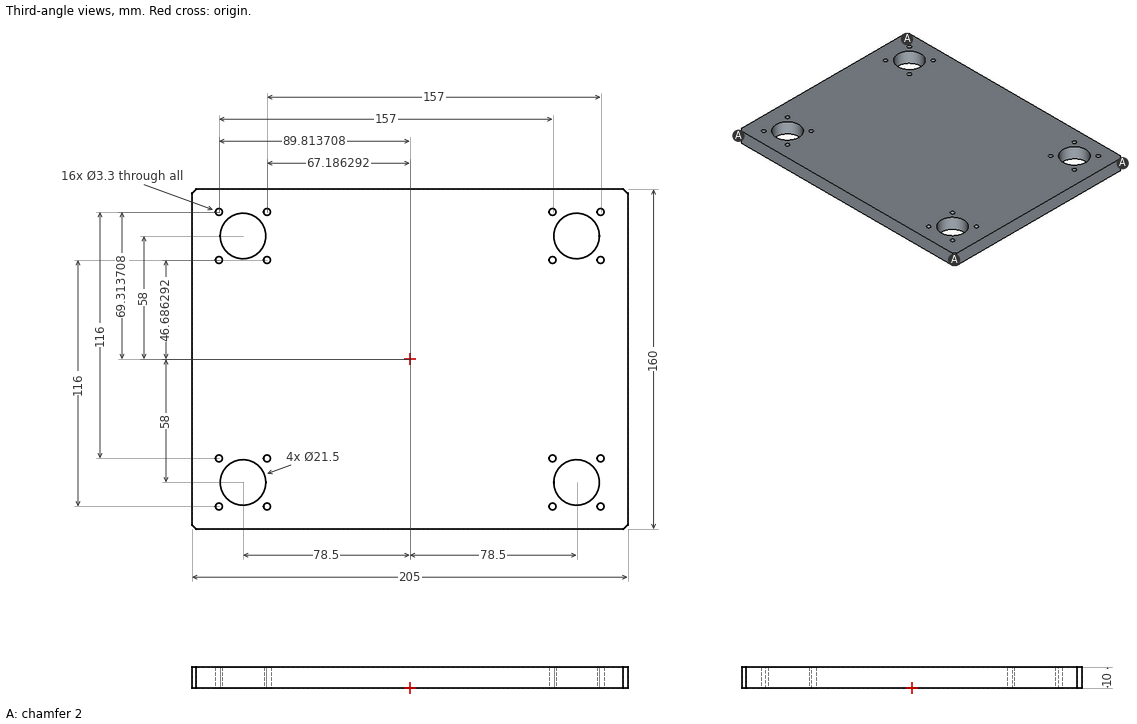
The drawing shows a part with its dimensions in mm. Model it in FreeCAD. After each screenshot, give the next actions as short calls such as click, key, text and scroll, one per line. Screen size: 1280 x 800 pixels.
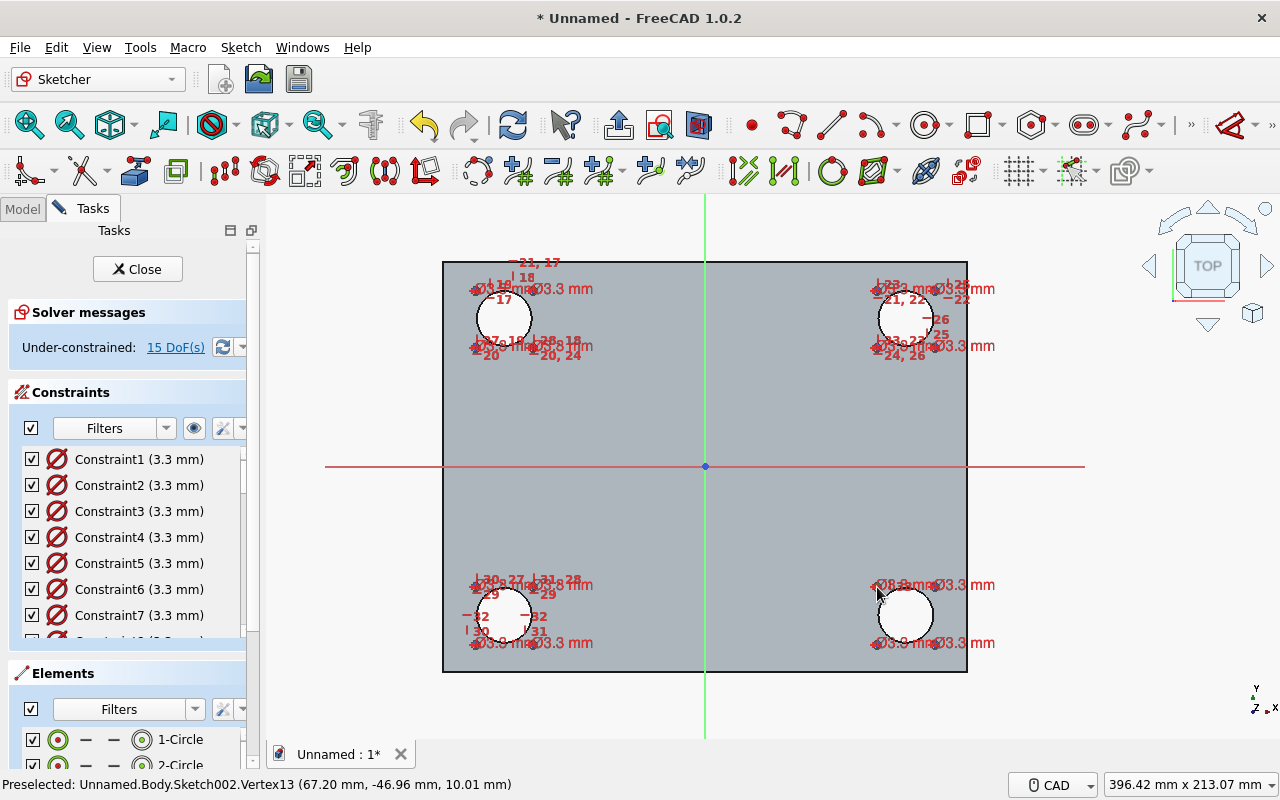
key(h)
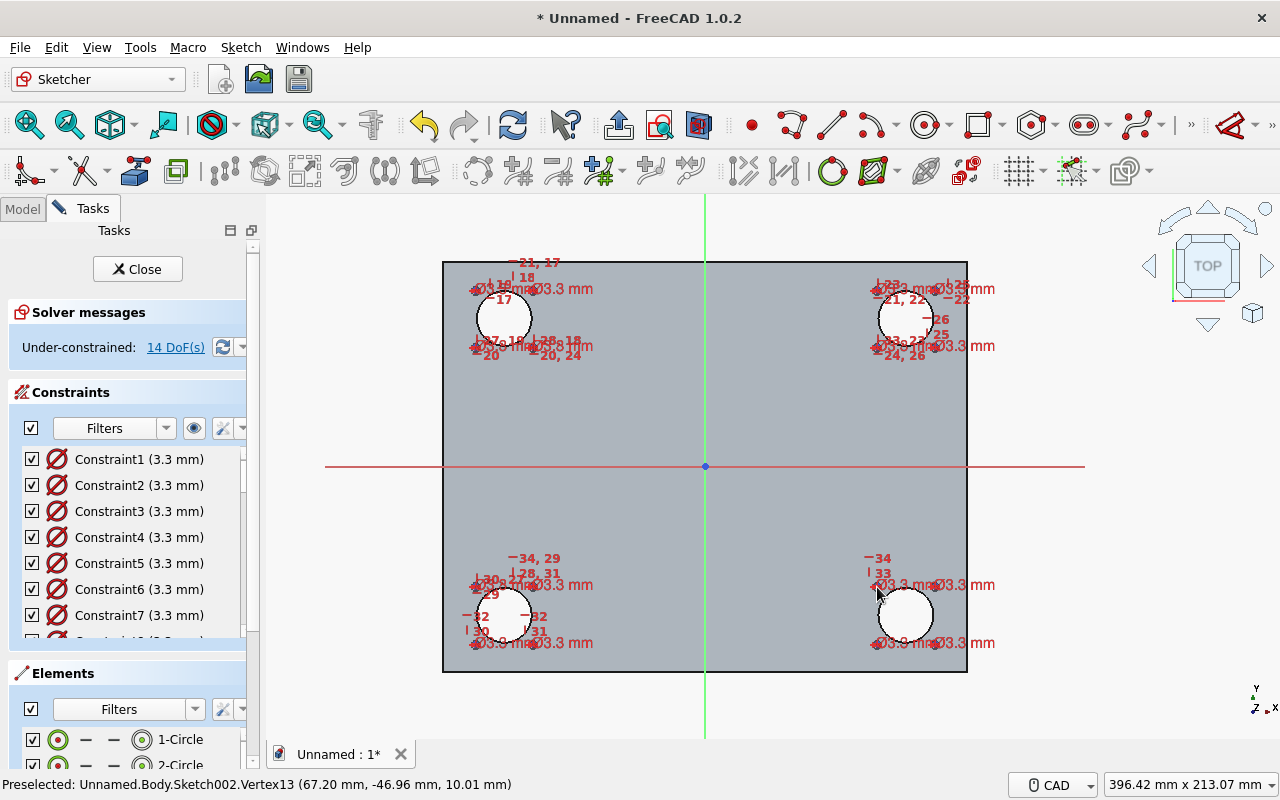
click(935, 348)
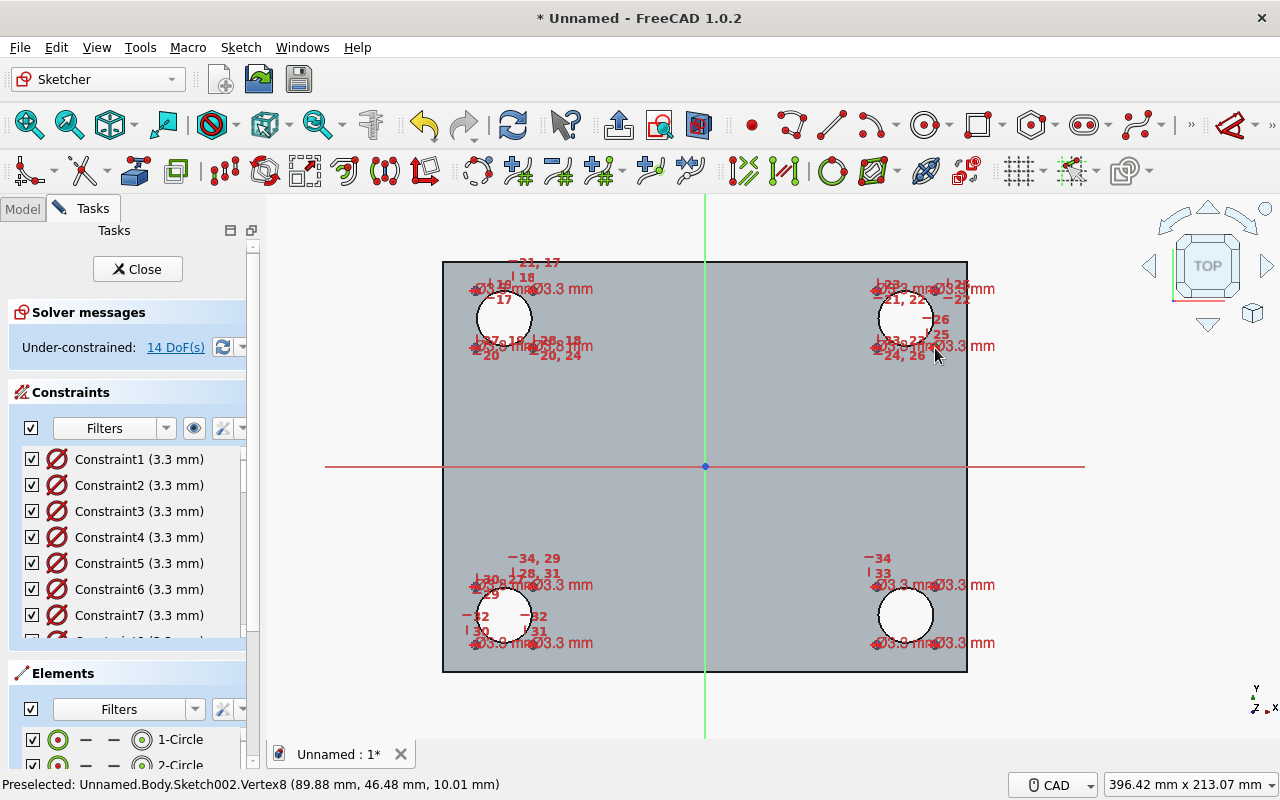
click(935, 587)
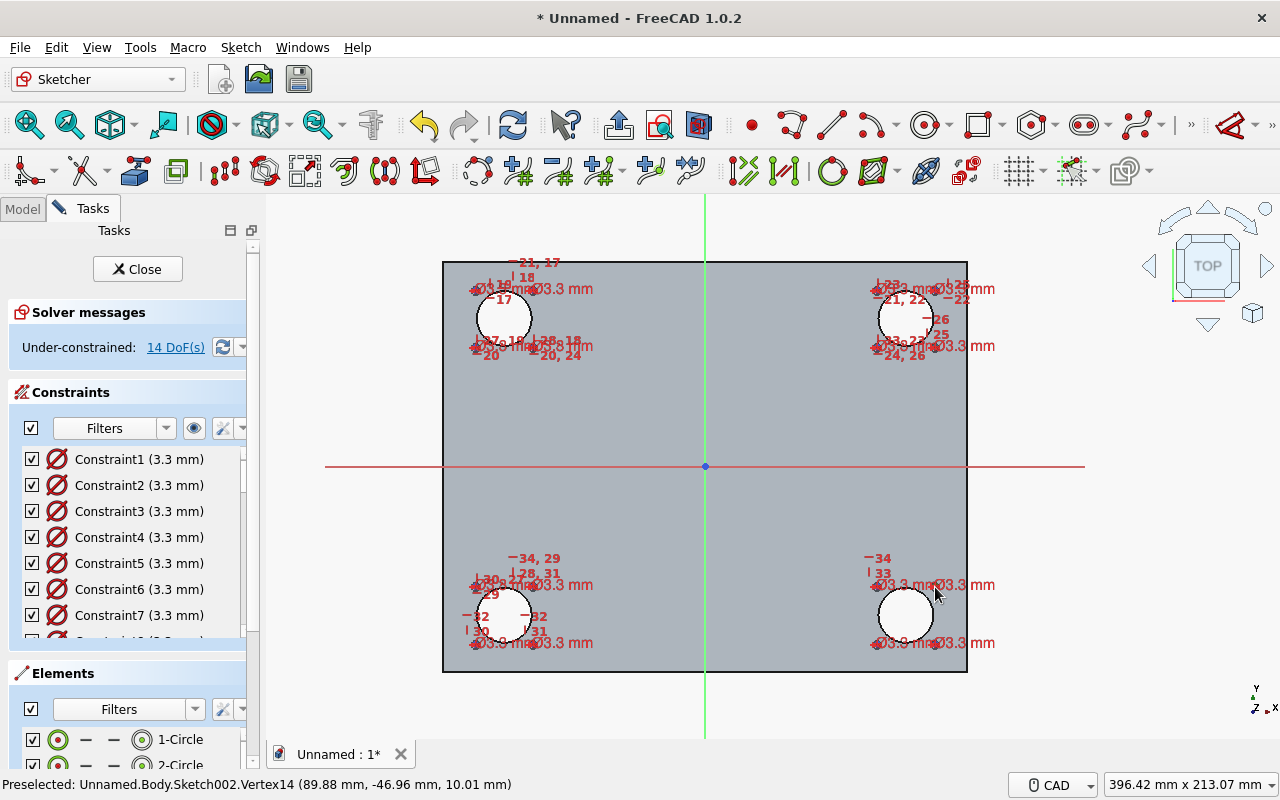
key(v)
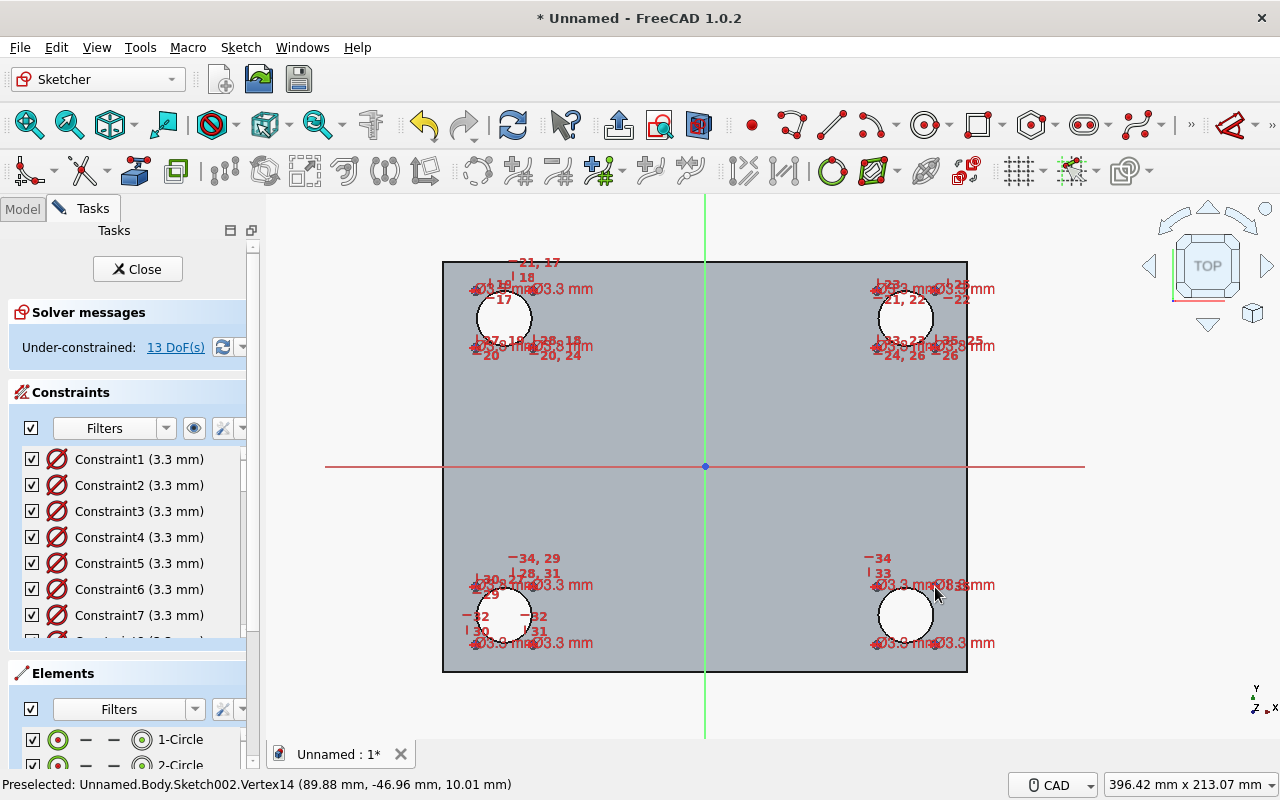
click(877, 587)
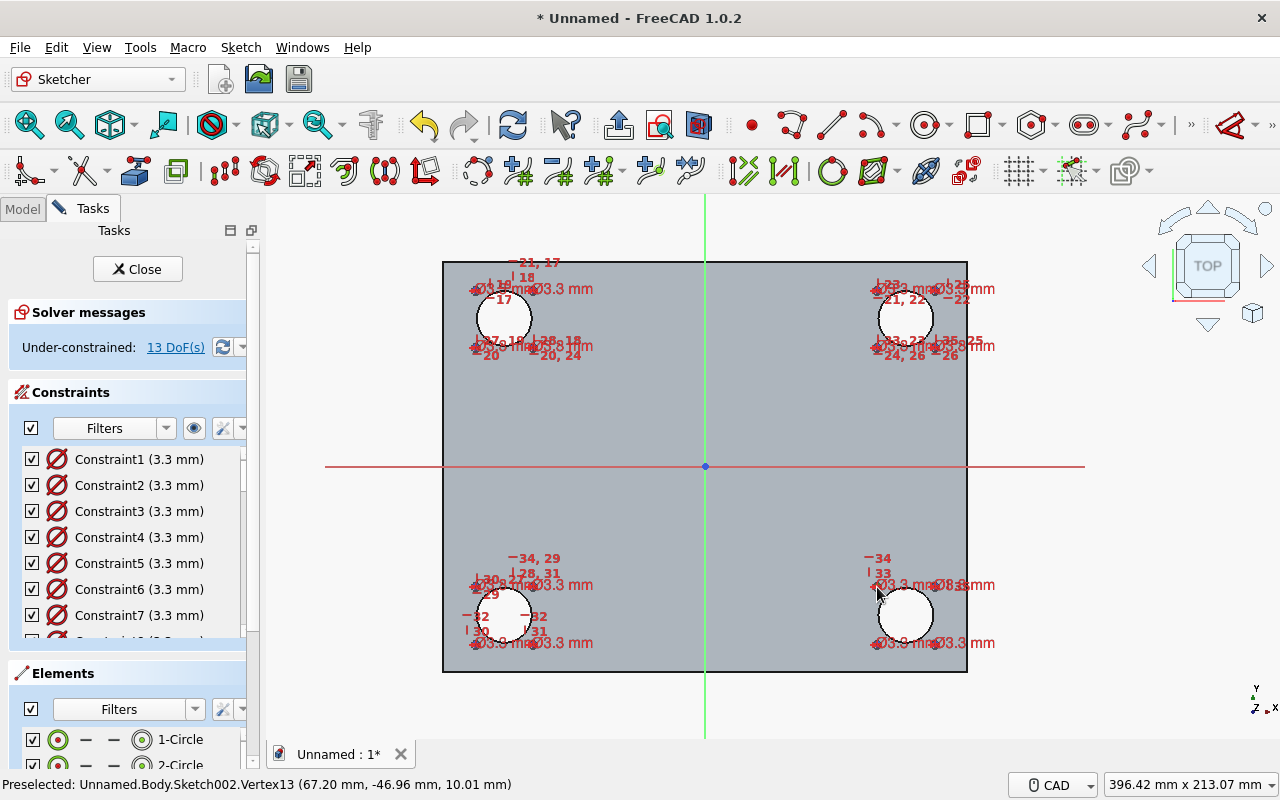
click(935, 587)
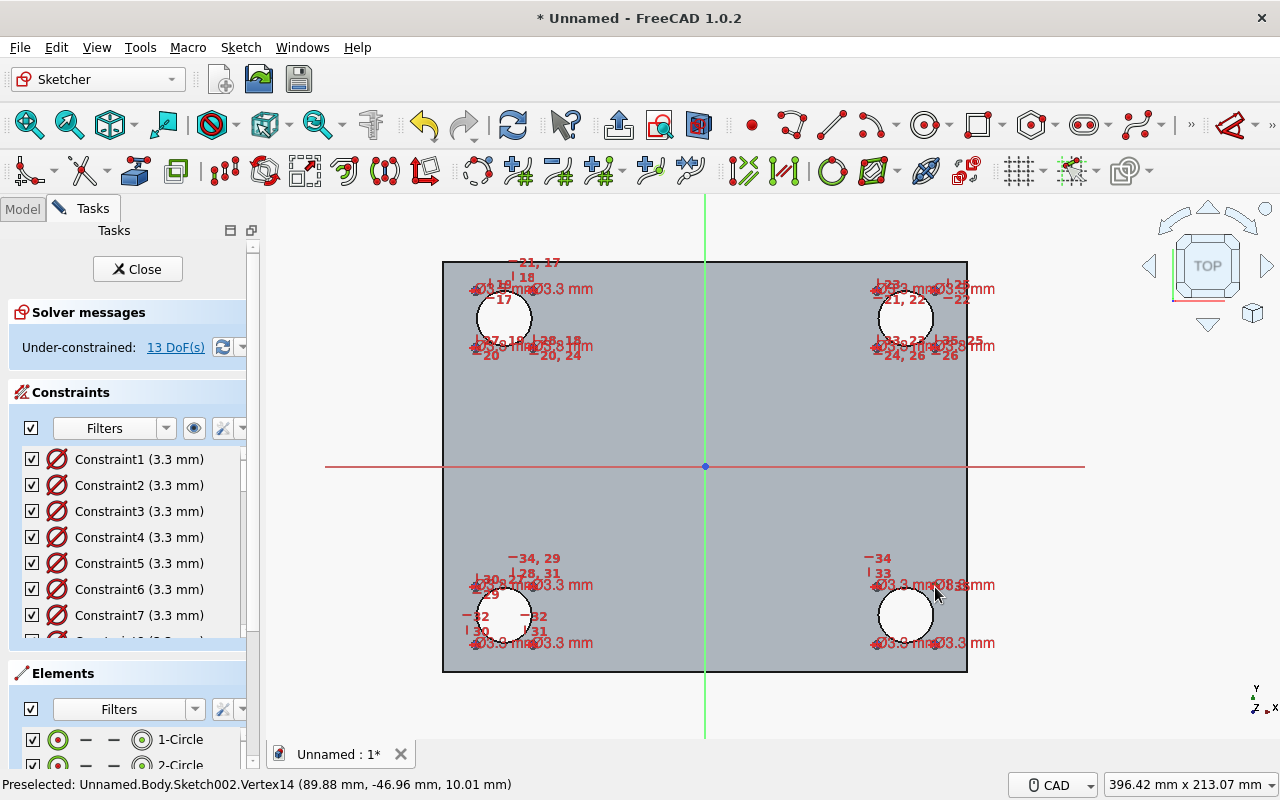
key(h)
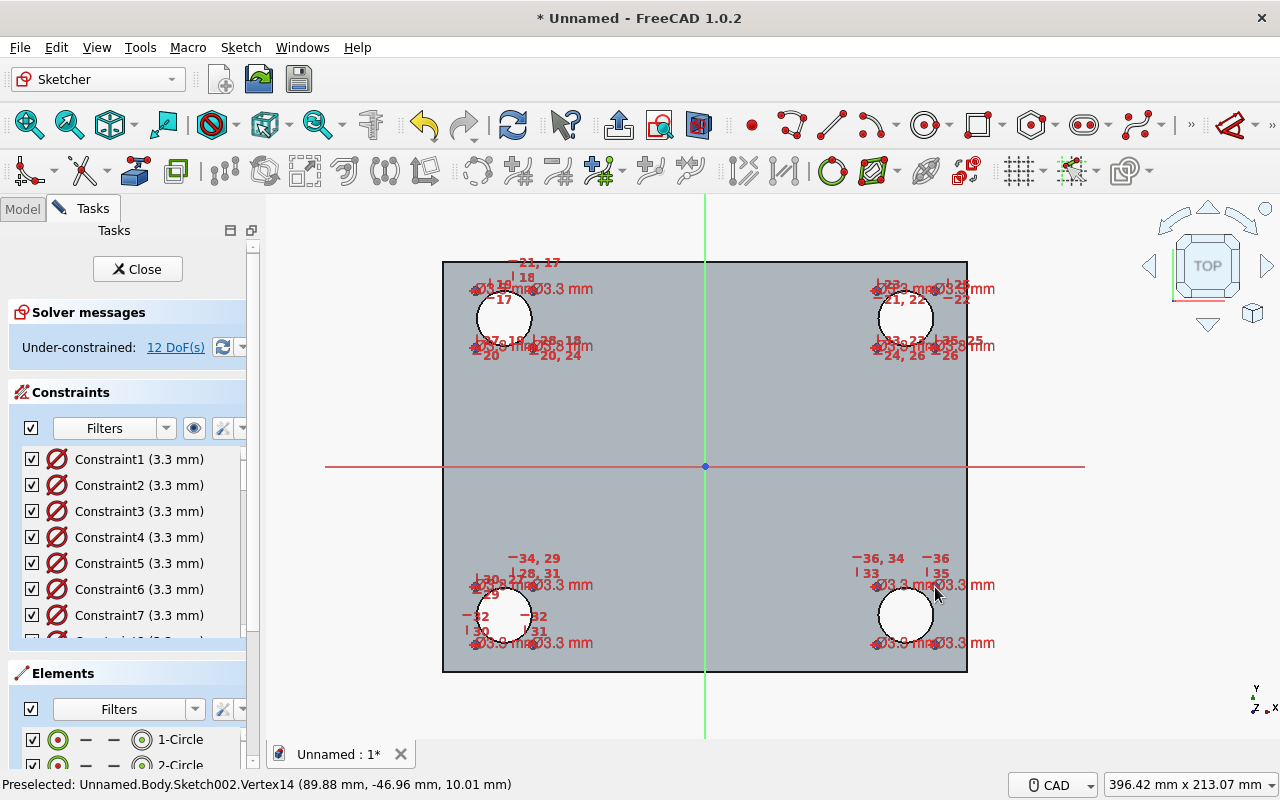
click(877, 587)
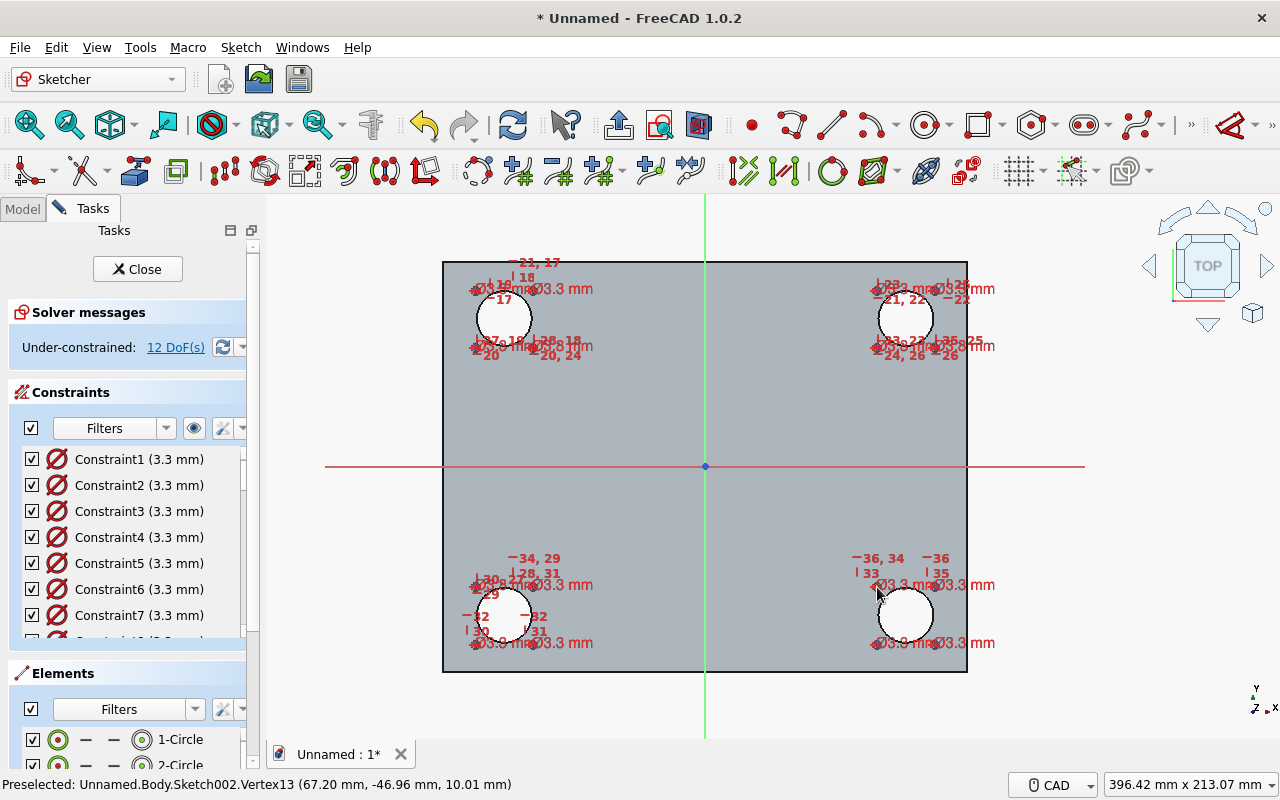
click(877, 645)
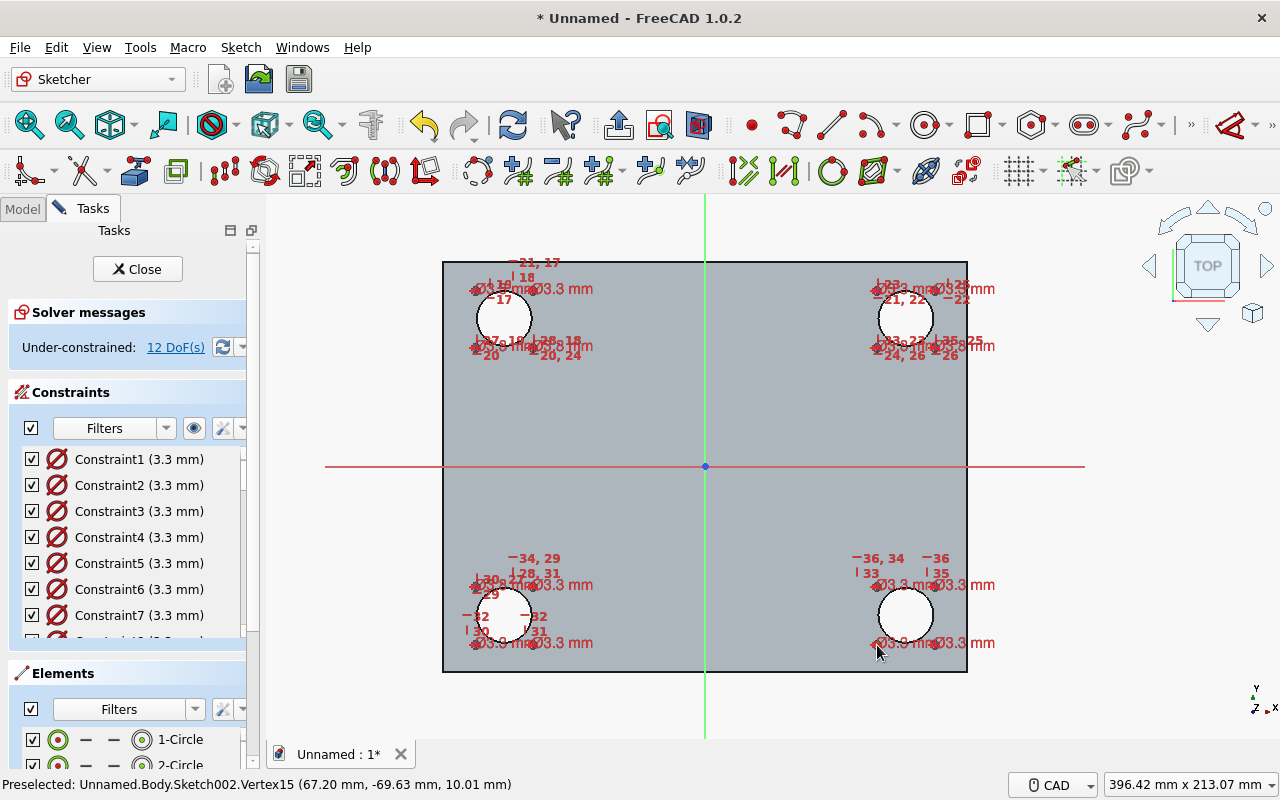
key(v)